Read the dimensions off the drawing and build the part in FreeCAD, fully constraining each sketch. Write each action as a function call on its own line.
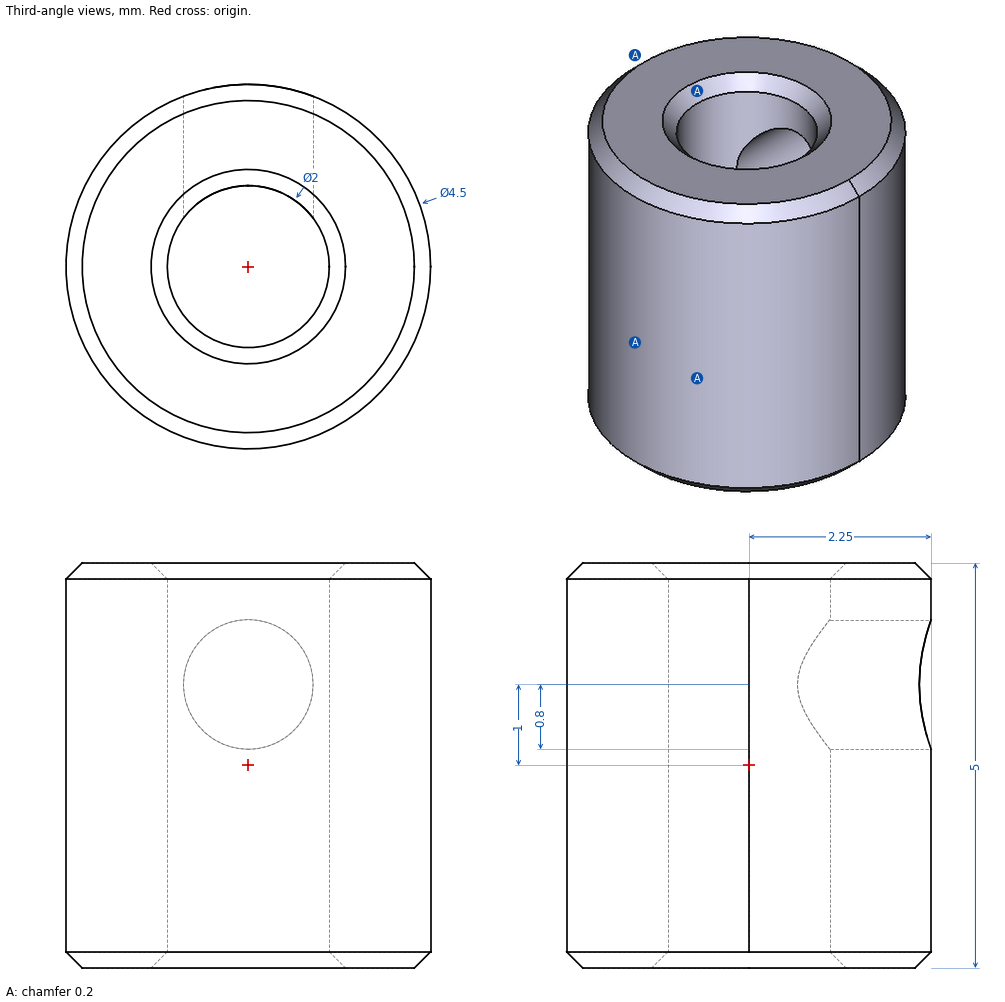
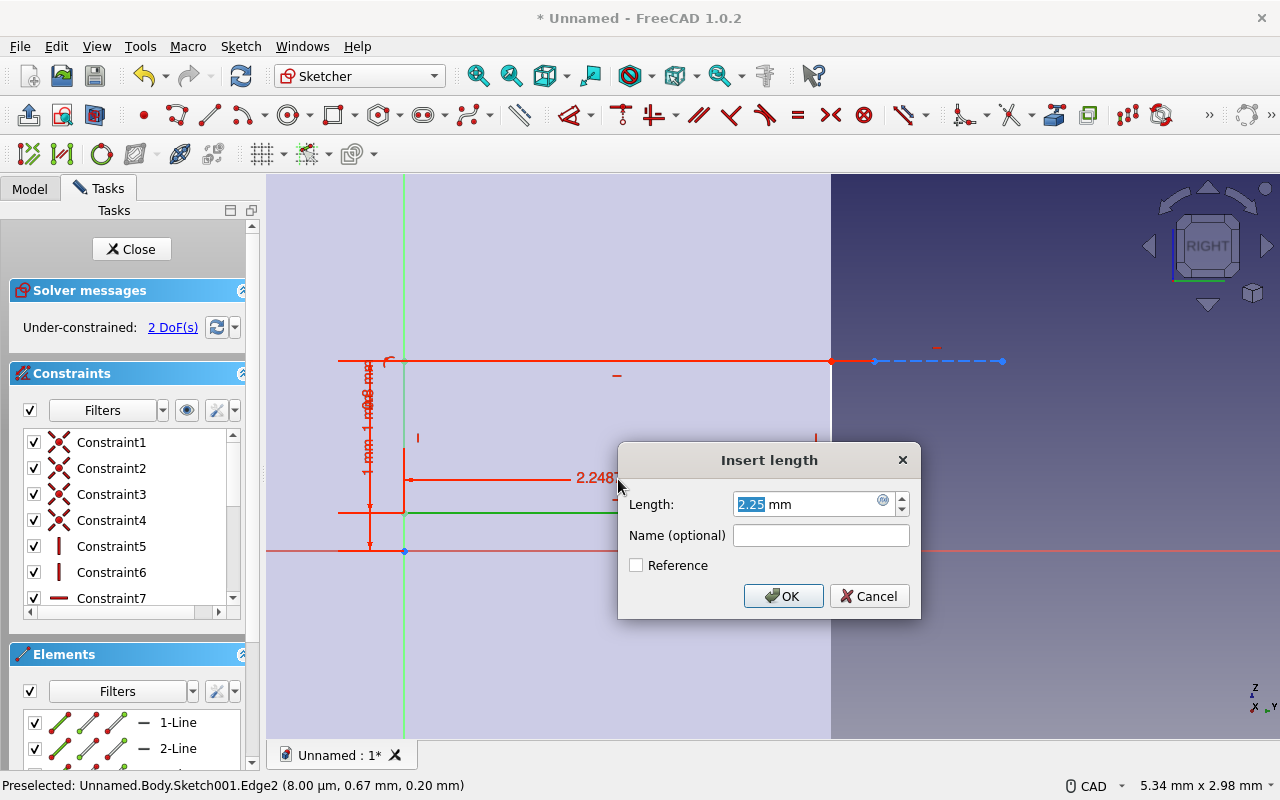
text(2.25)
key(Return)
key(Escape)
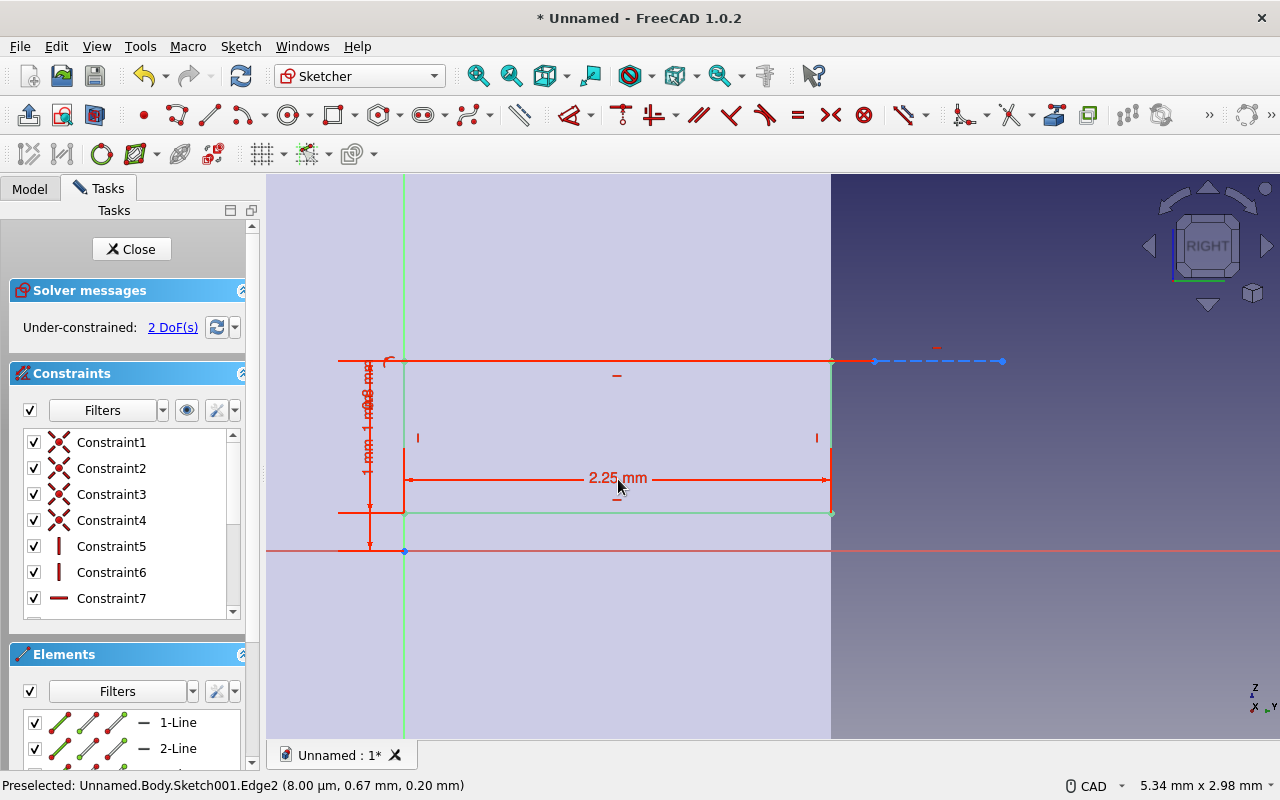
click(132, 249)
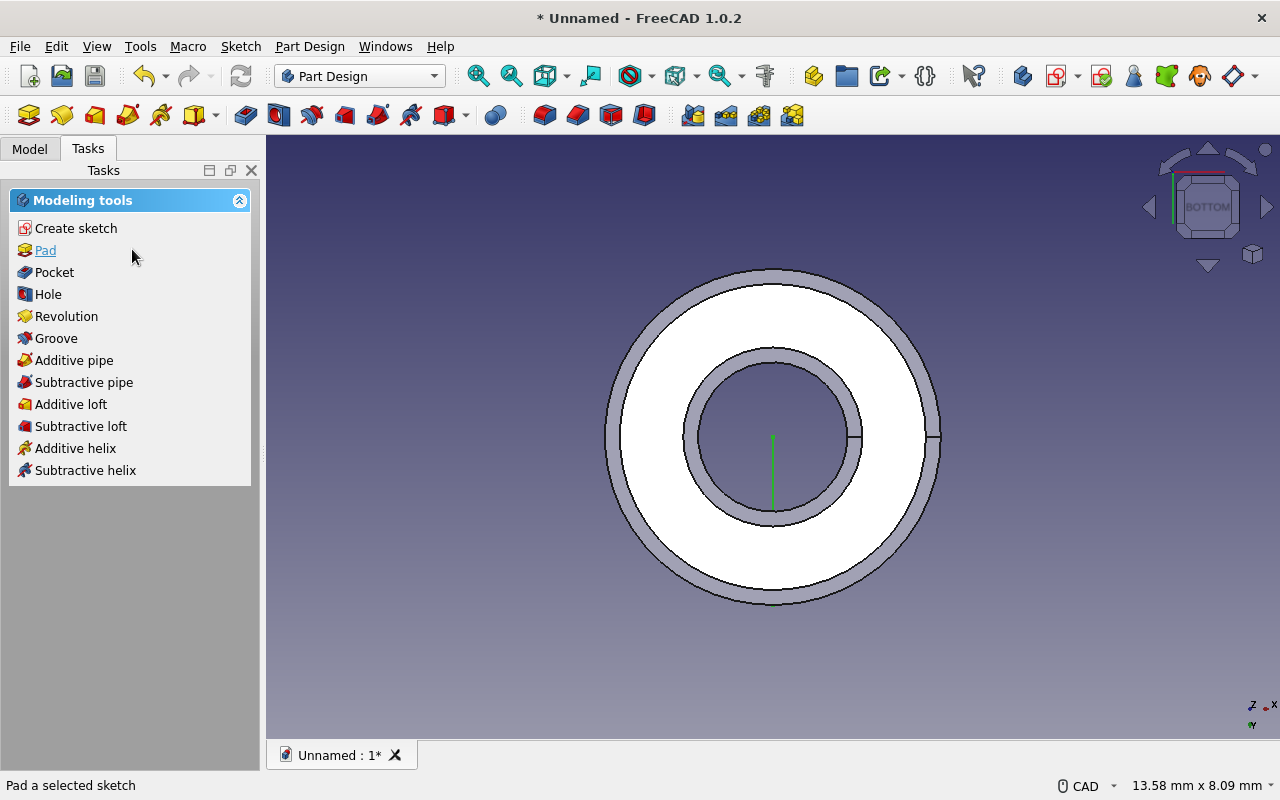
click(312, 116)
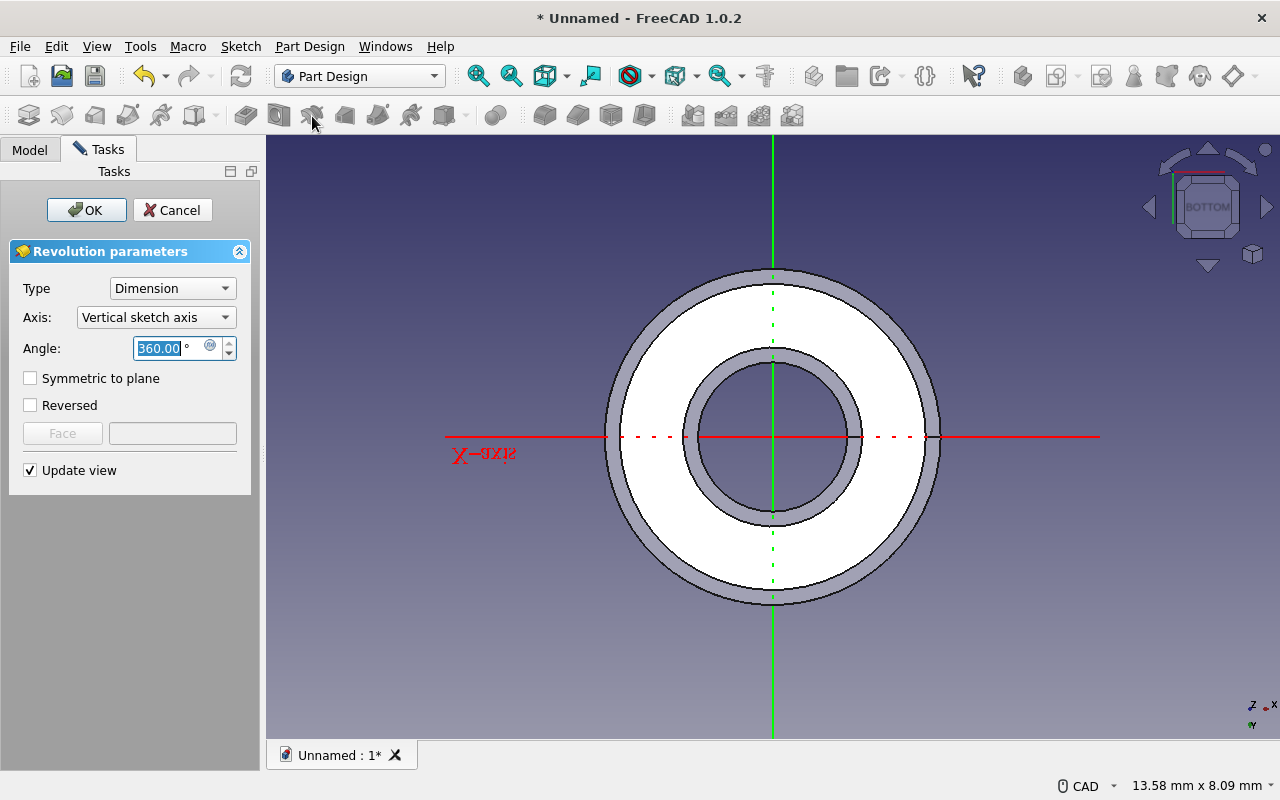
click(157, 318)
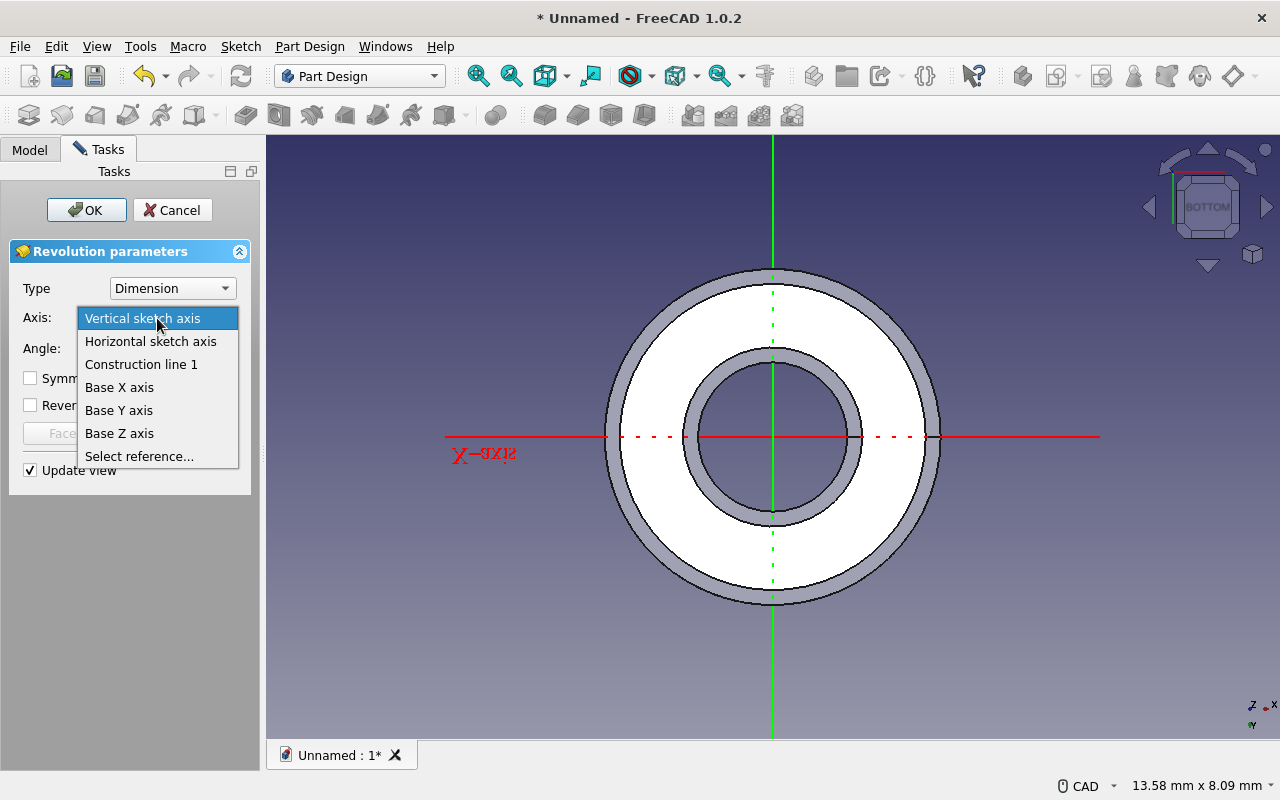
click(156, 364)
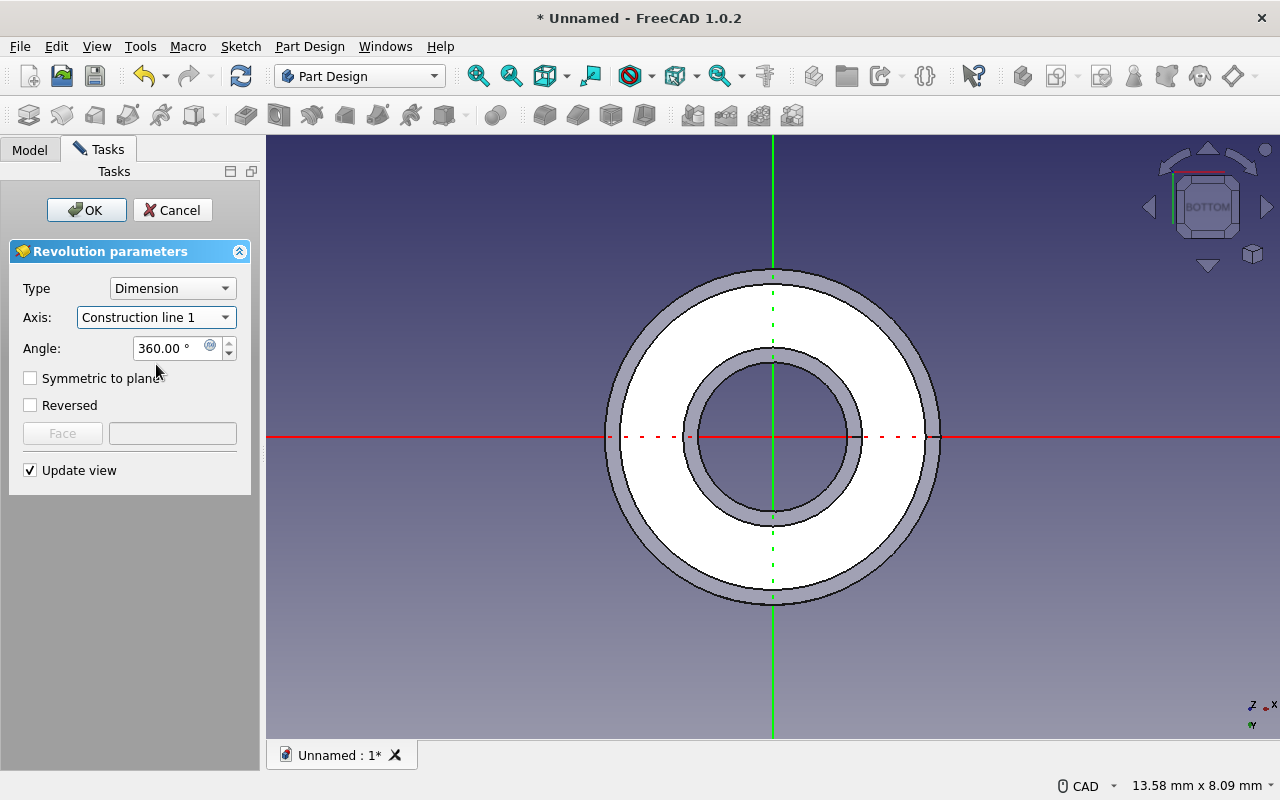
click(87, 210)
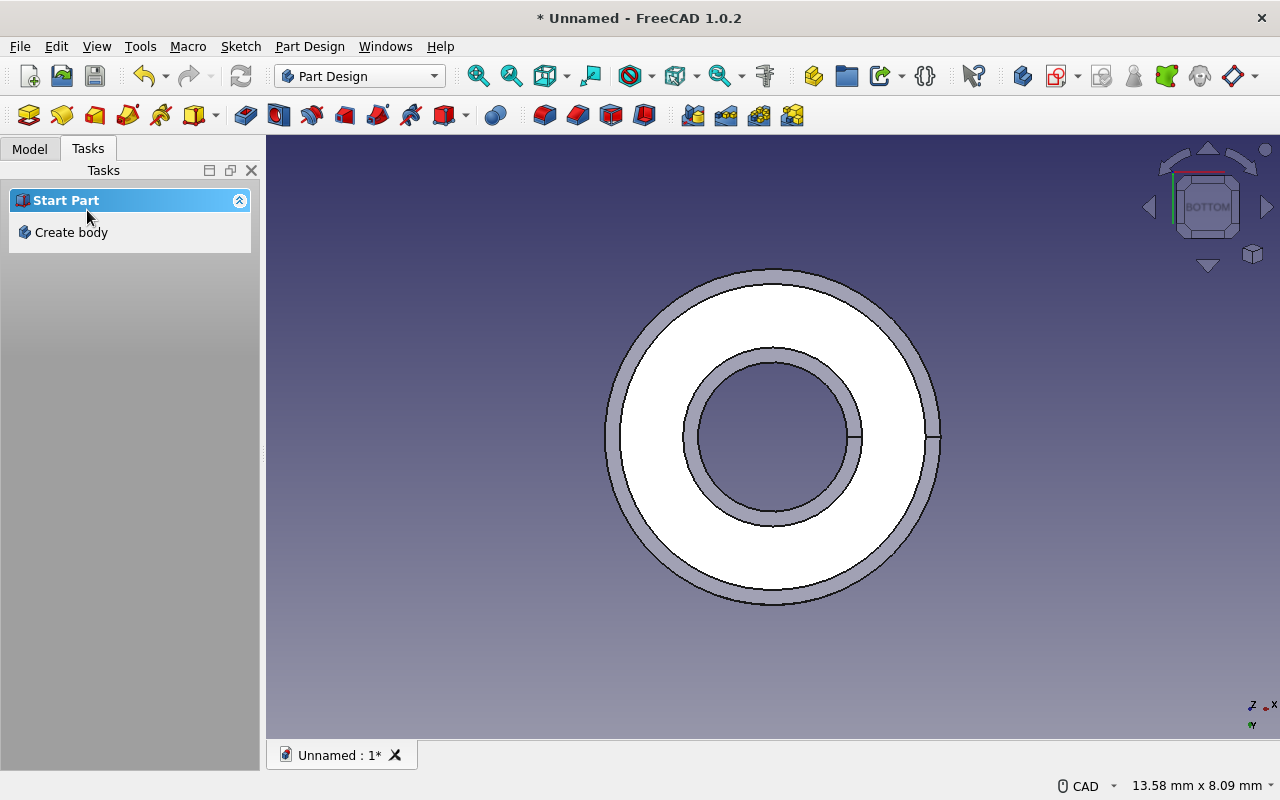
key(0)